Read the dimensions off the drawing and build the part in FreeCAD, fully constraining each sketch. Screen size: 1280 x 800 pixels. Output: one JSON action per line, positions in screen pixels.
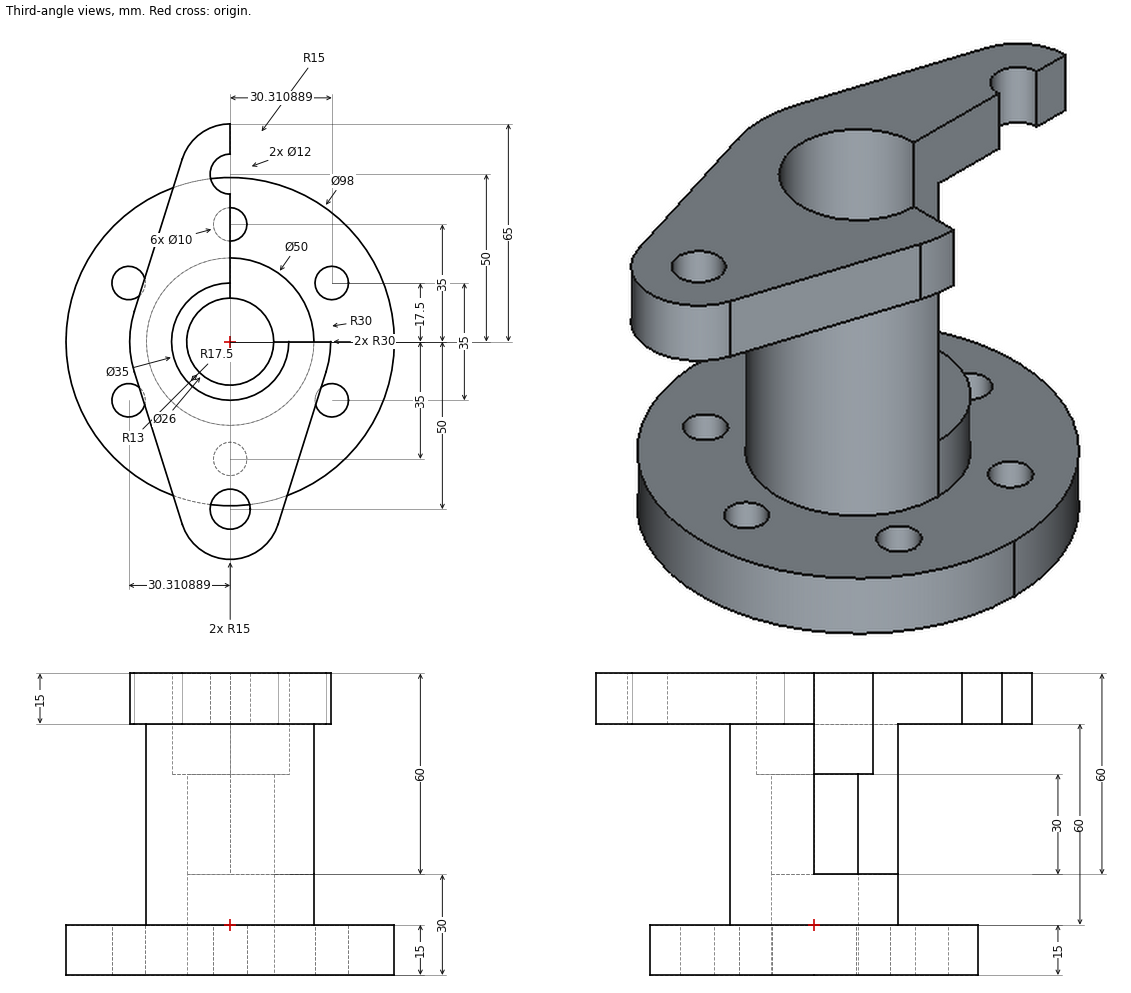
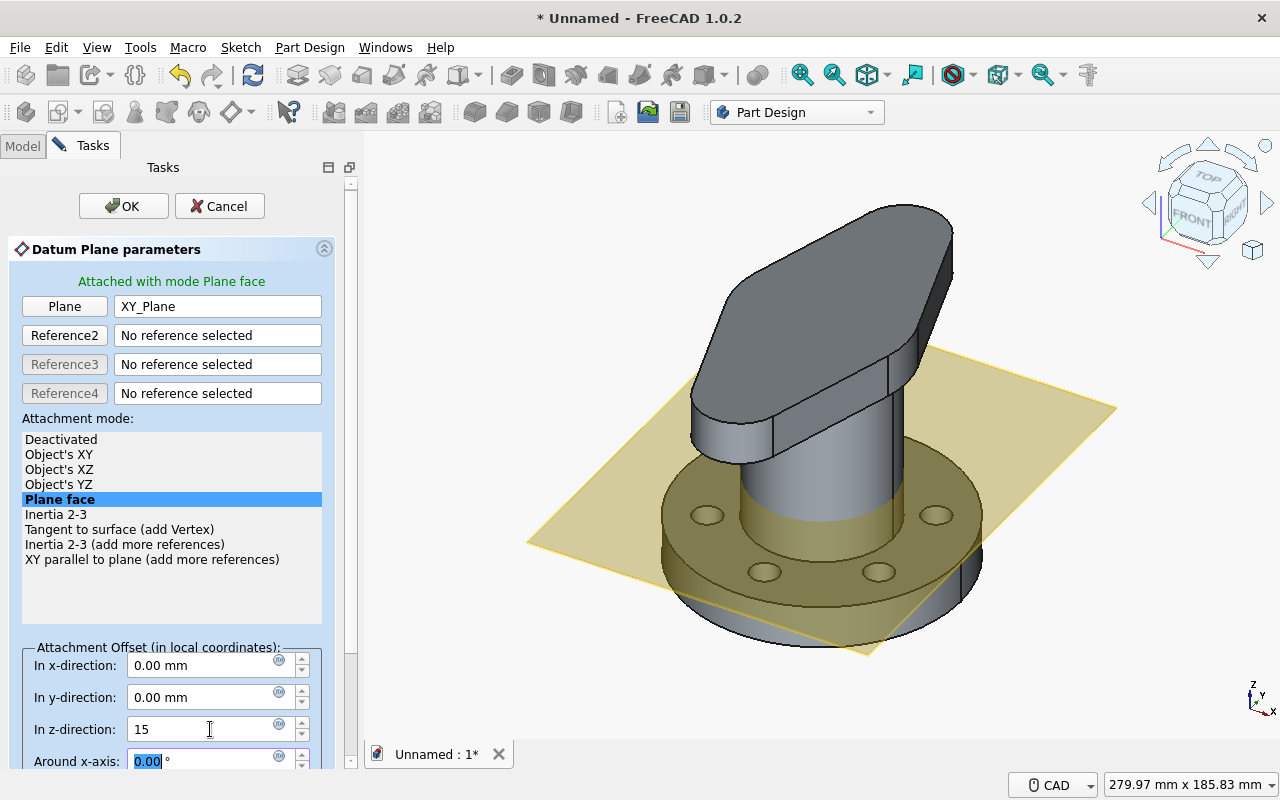
{"action": "left_click", "coordinate": [124, 206]}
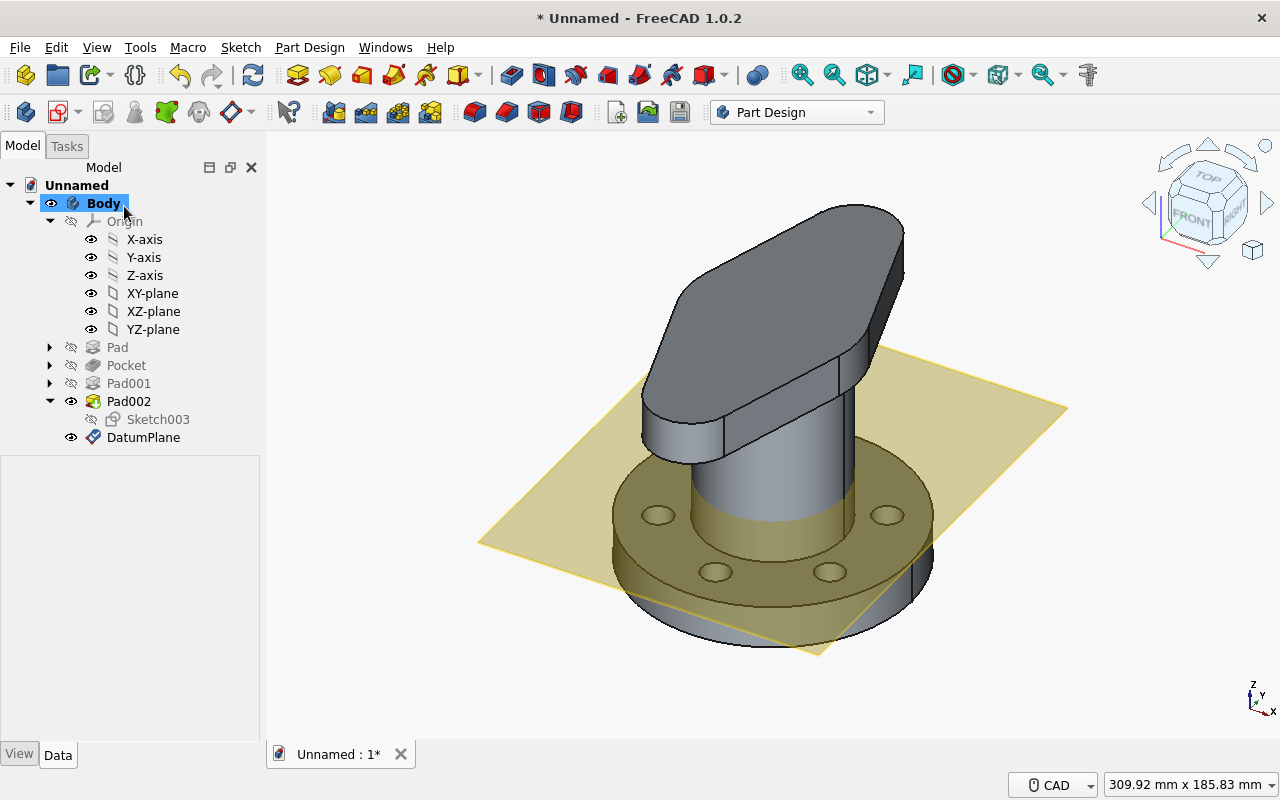
{"action": "left_click", "coordinate": [116, 437]}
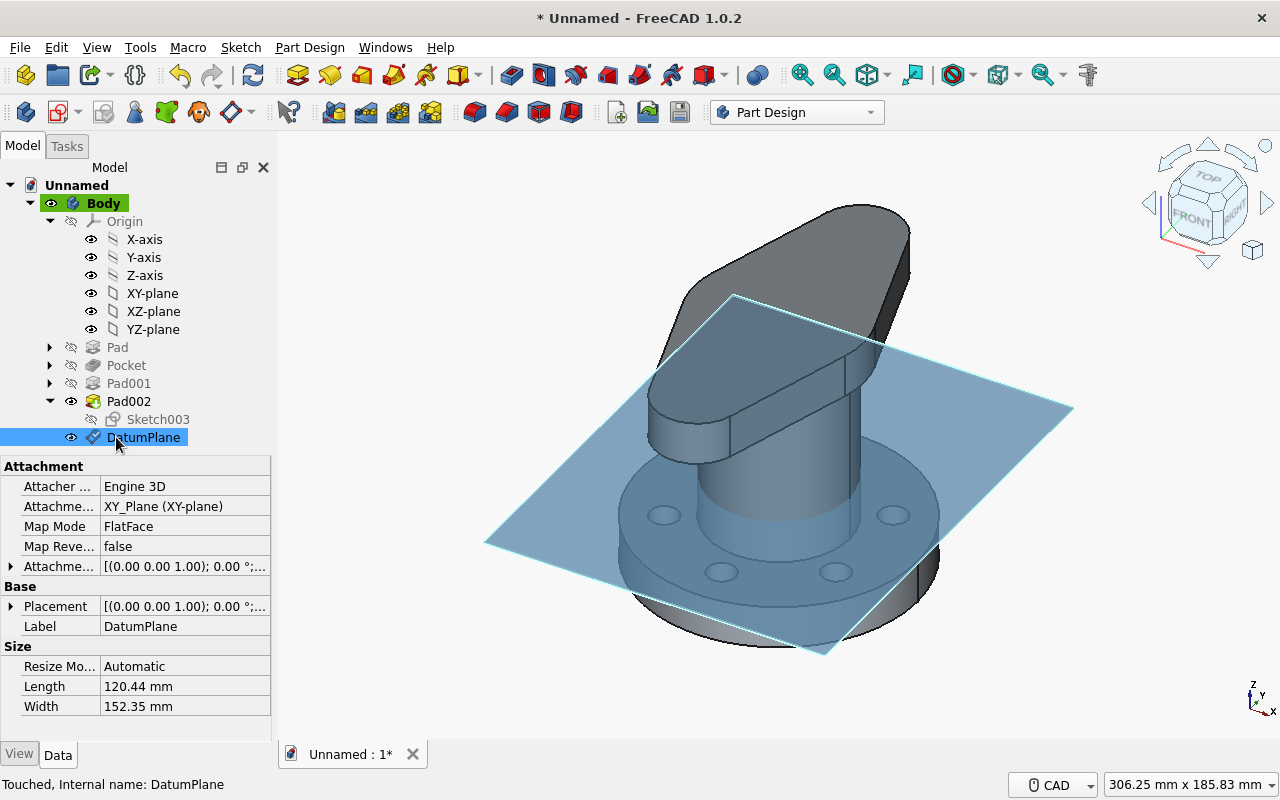
{"action": "left_click", "coordinate": [58, 112]}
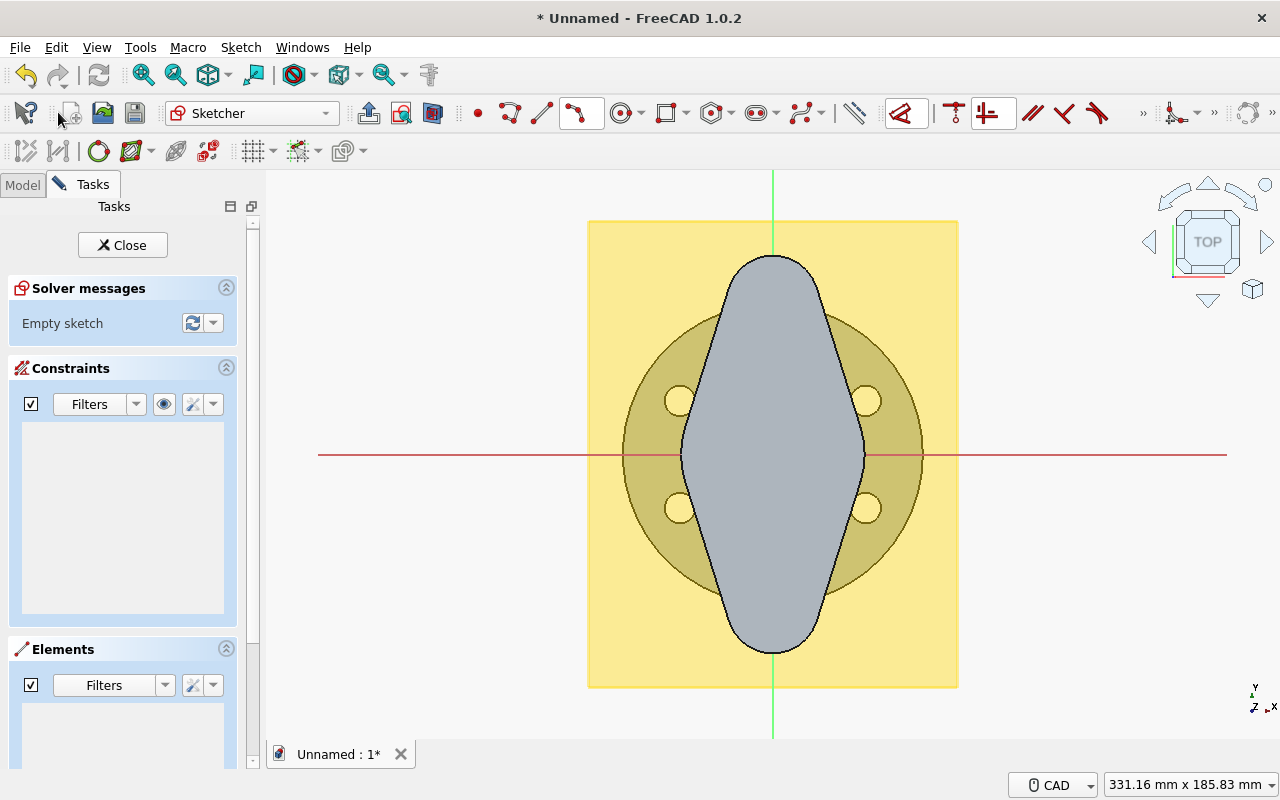
{"action": "left_click", "coordinate": [434, 114]}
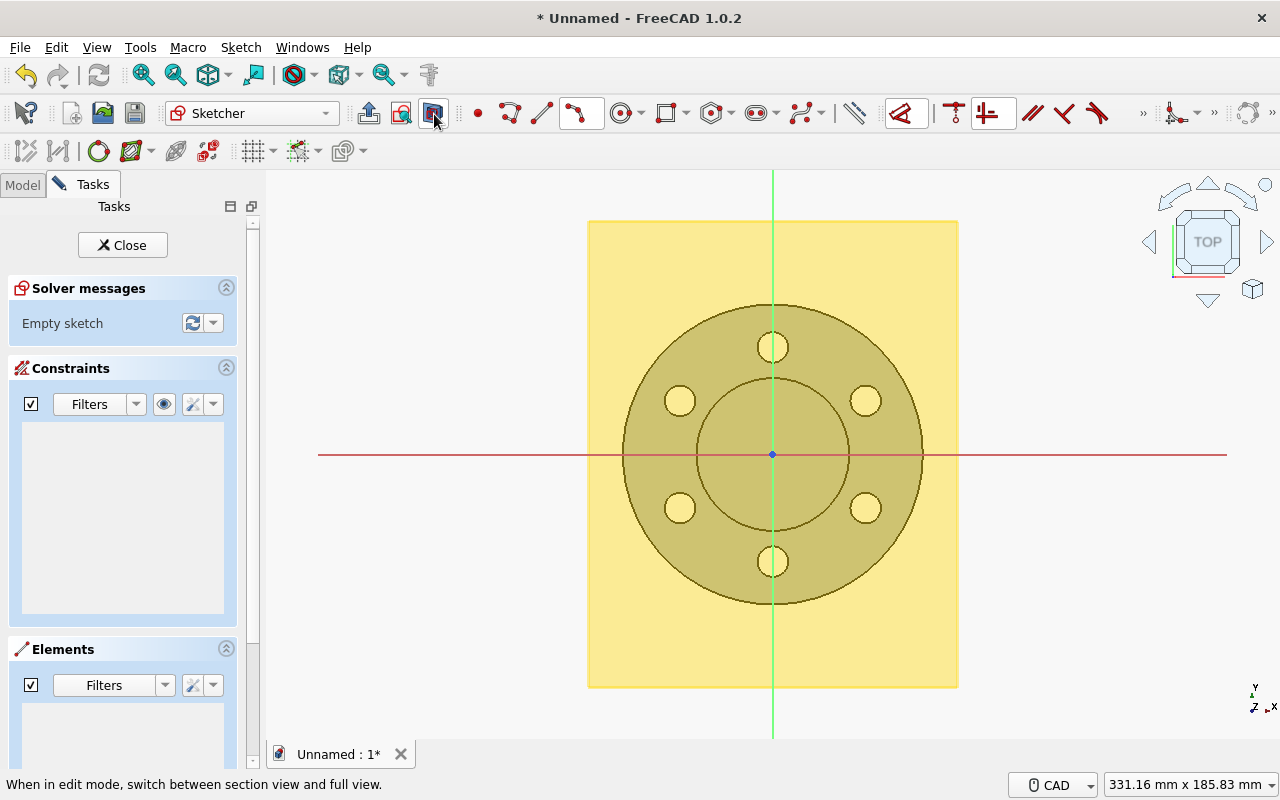
{"action": "scroll", "coordinate": [958, 234], "scroll_direction": "up", "scroll_amount": 3}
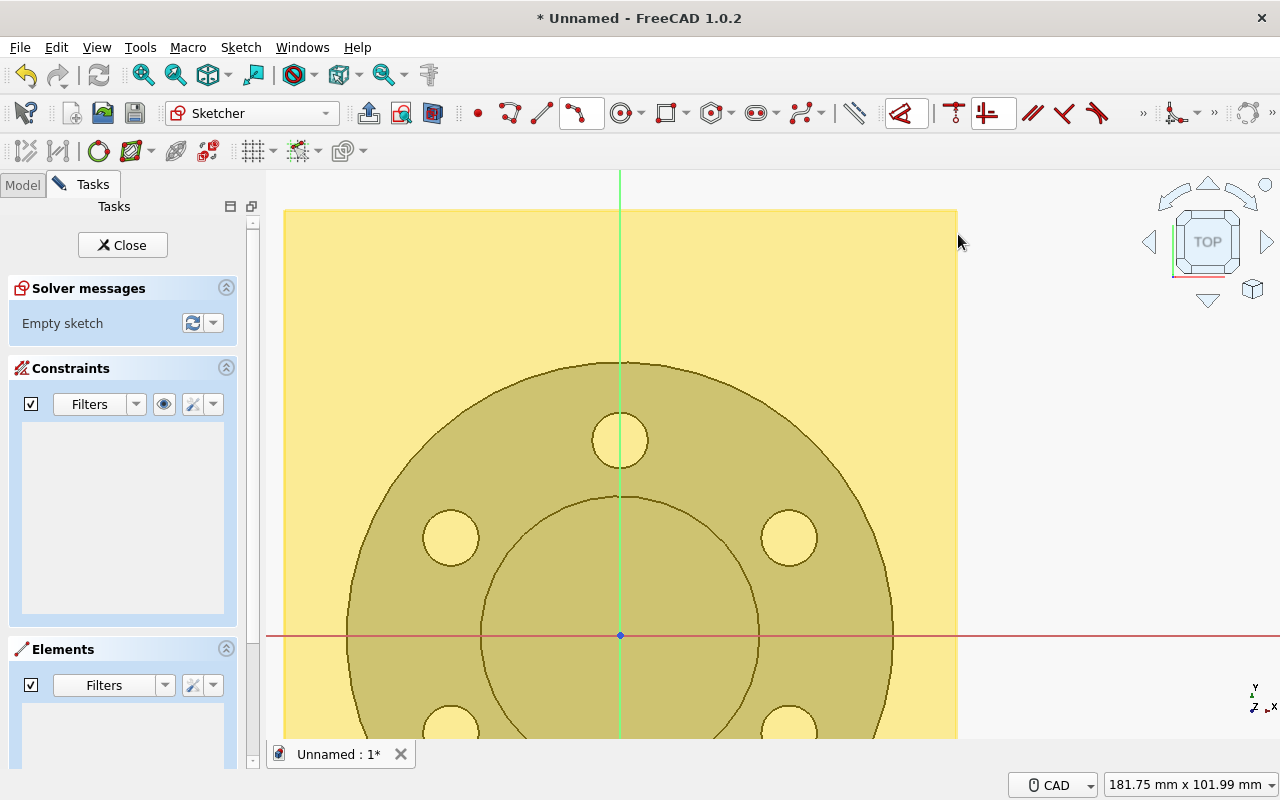
{"action": "left_click", "coordinate": [510, 114]}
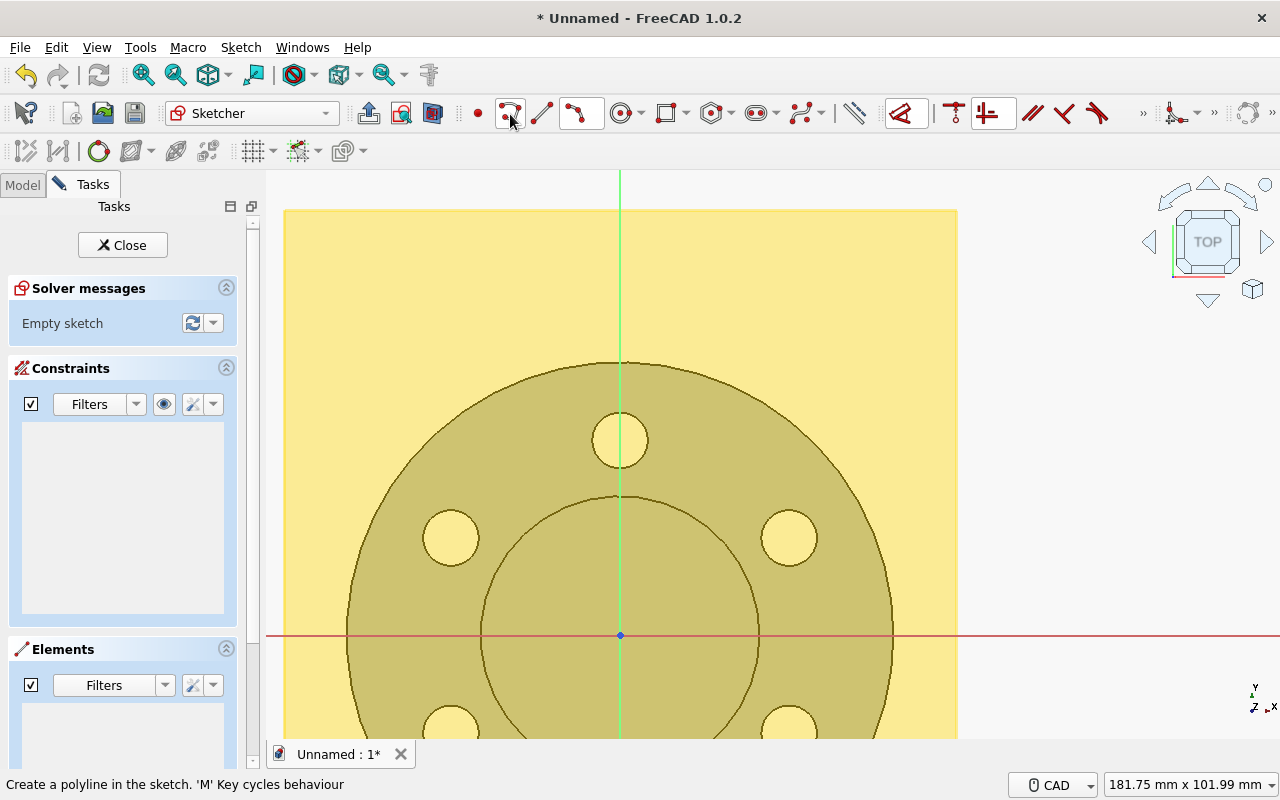
{"action": "left_click", "coordinate": [620, 273]}
{"action": "left_click", "coordinate": [620, 636]}
{"action": "left_click", "coordinate": [787, 627]}
{"action": "right_click", "coordinate": [787, 627]}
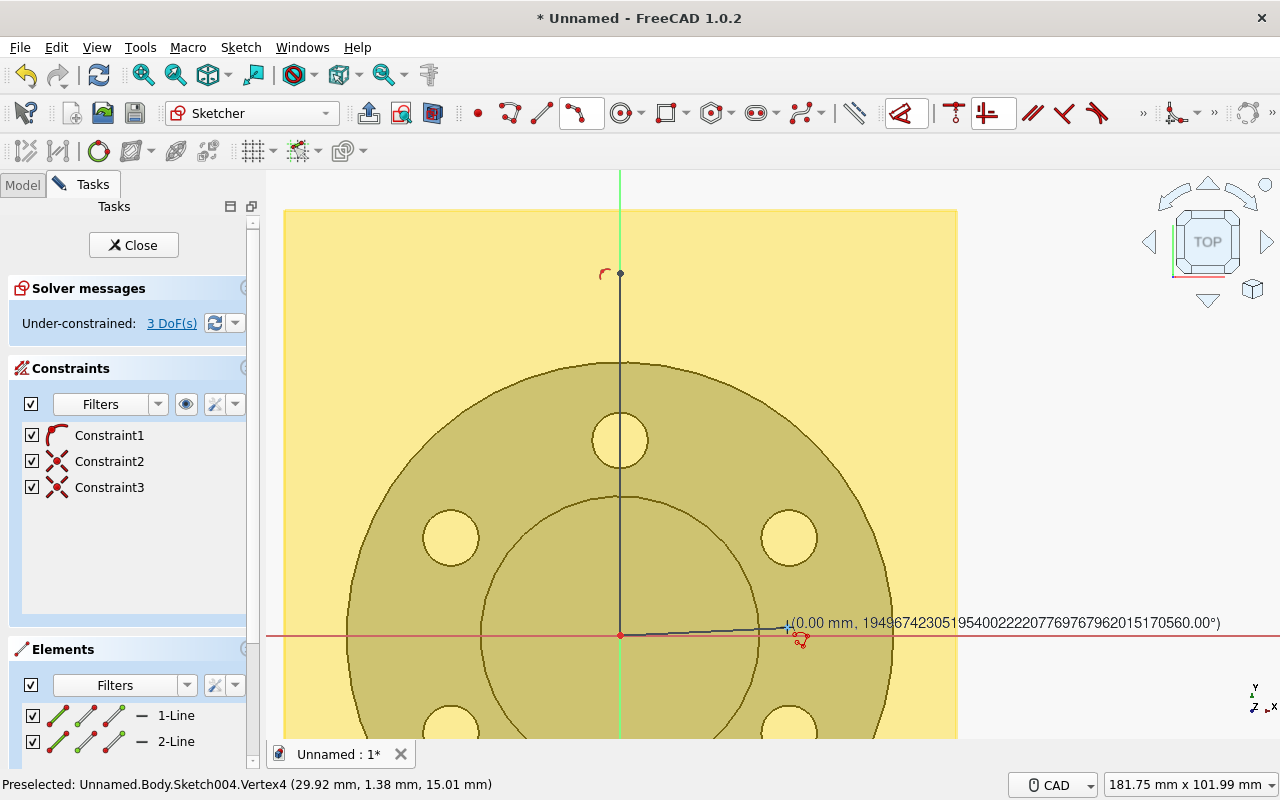
{"action": "left_click", "coordinate": [542, 114]}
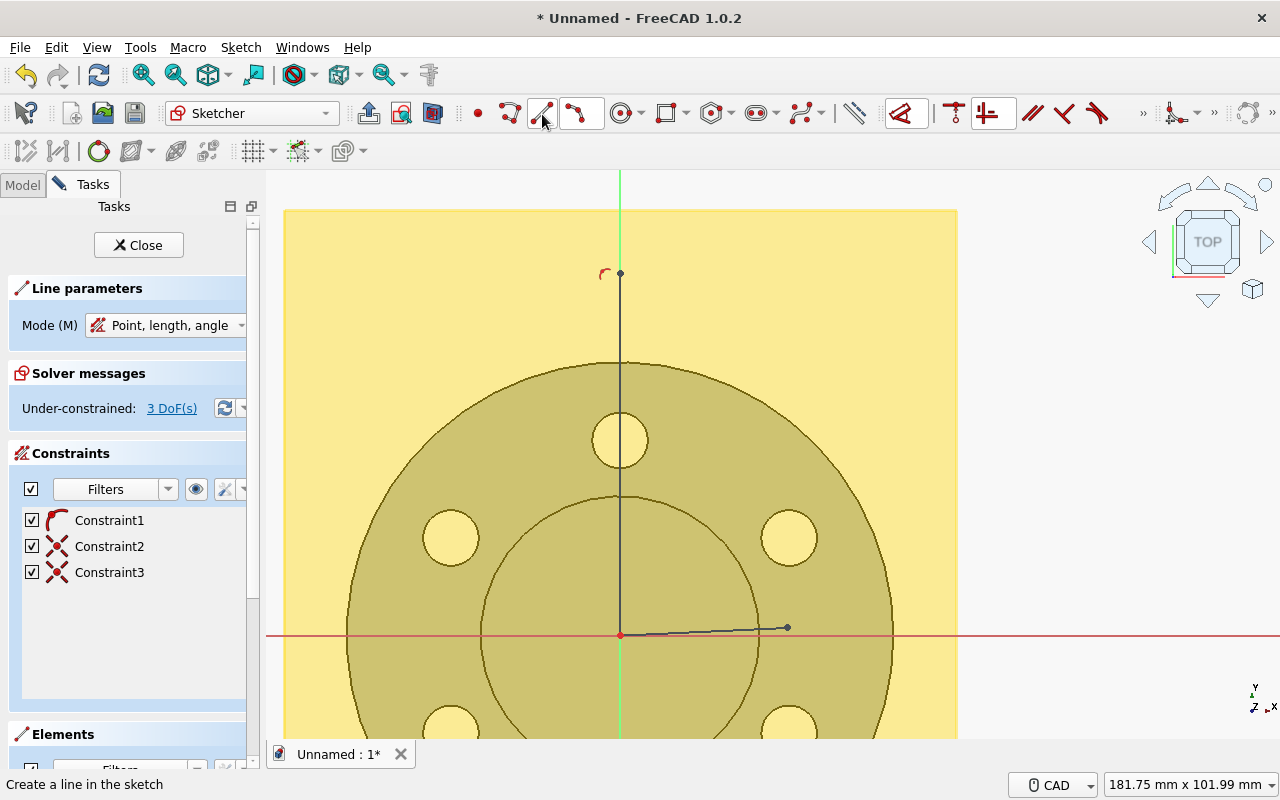
{"action": "left_click", "coordinate": [780, 585]}
{"action": "left_click", "coordinate": [700, 332]}